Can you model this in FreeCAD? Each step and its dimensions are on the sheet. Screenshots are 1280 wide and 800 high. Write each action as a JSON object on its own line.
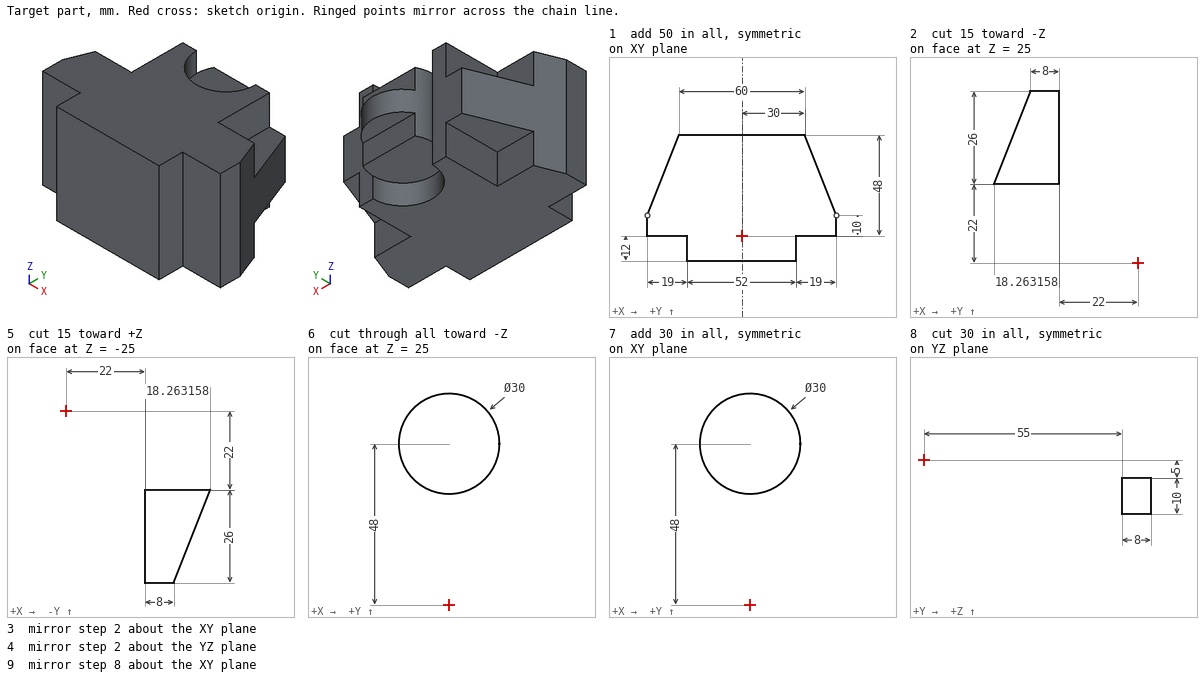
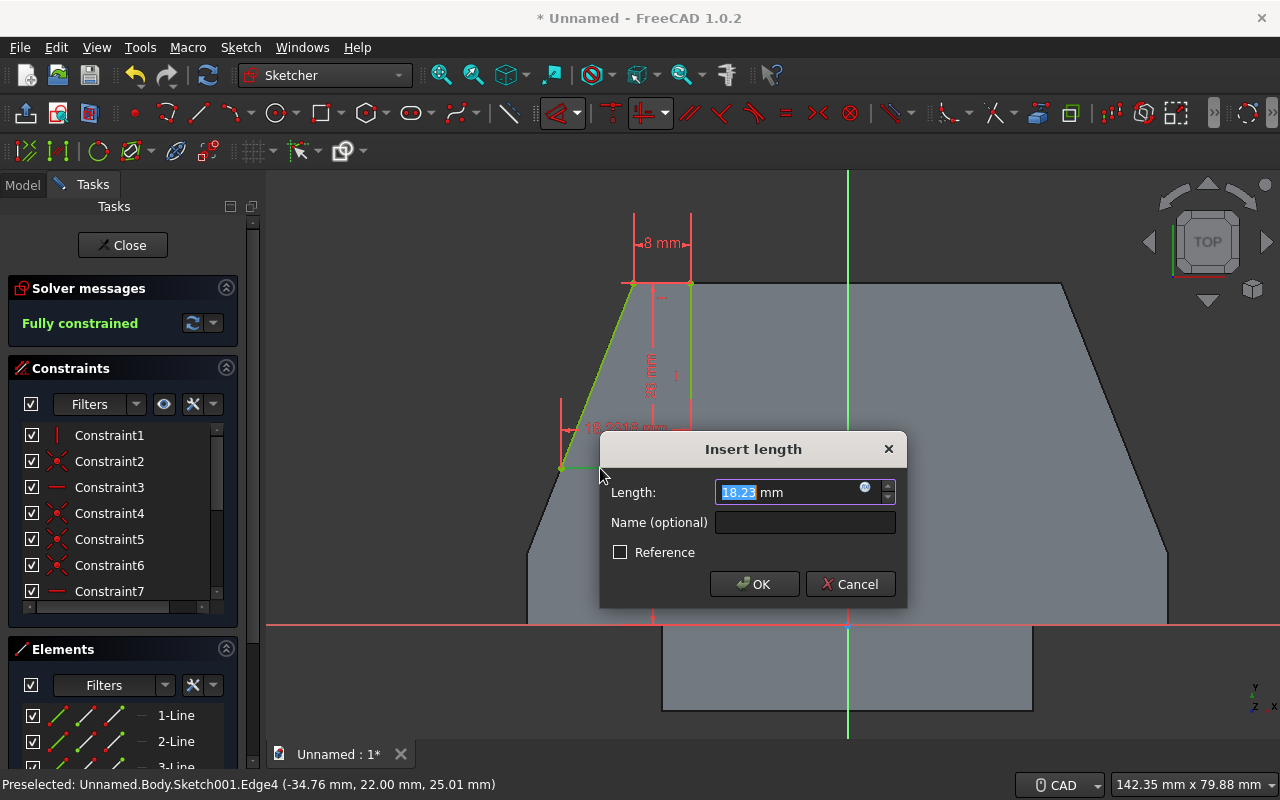
{"action": "type", "text": "18.263158"}
{"action": "key", "text": "Return"}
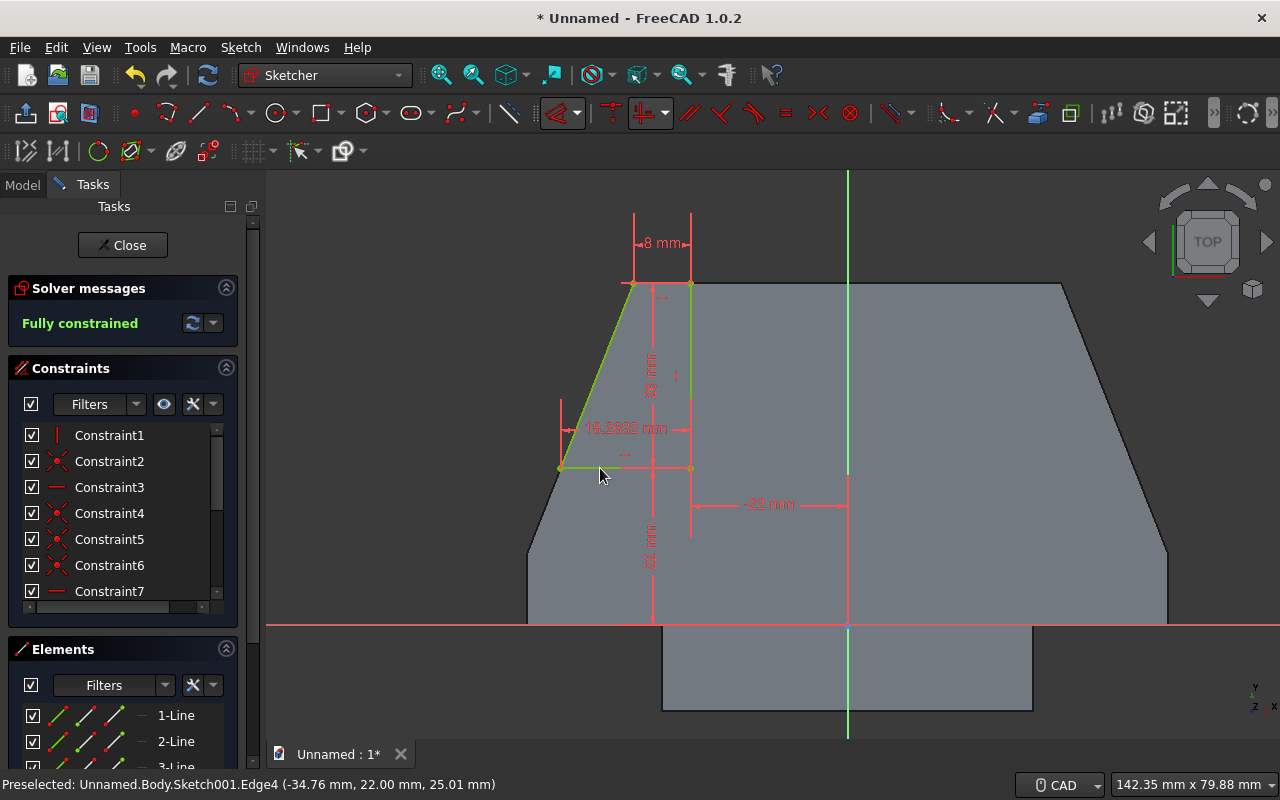
{"action": "left_click", "coordinate": [123, 245]}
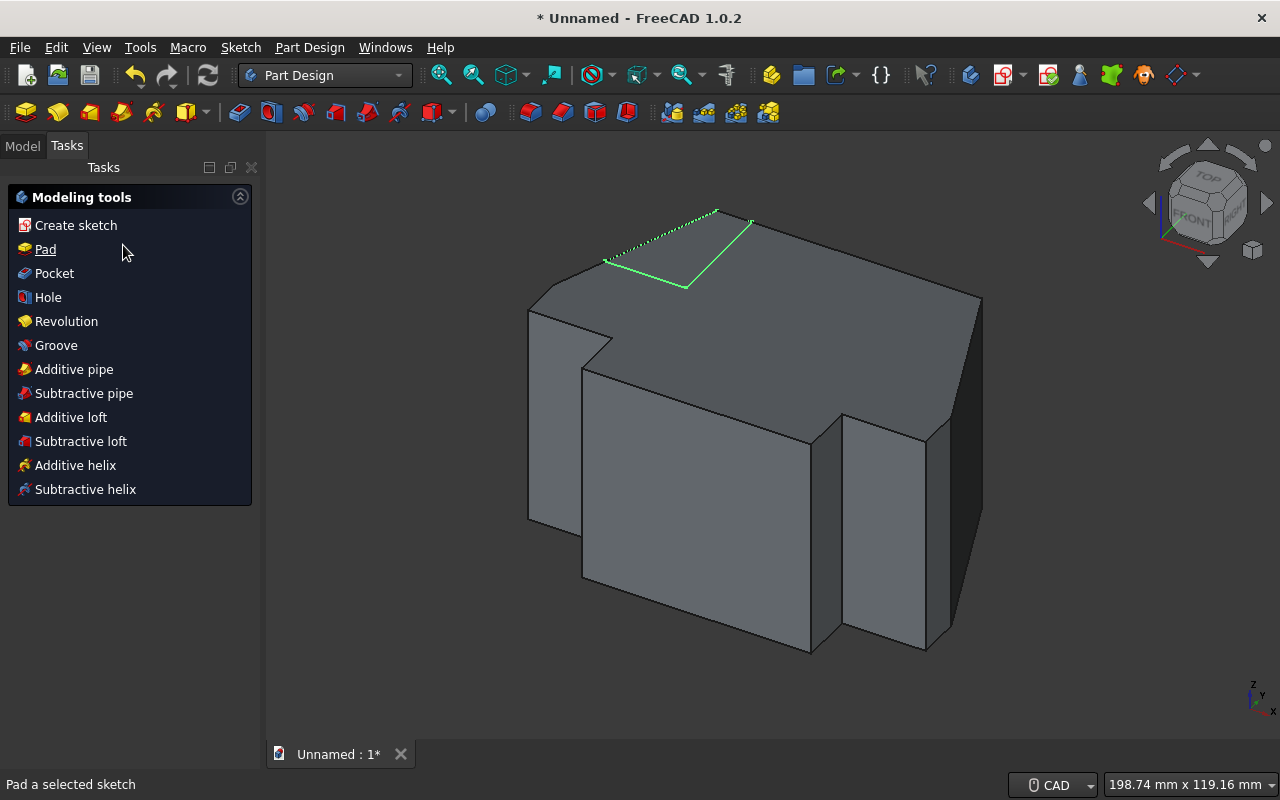
{"action": "left_click", "coordinate": [240, 112]}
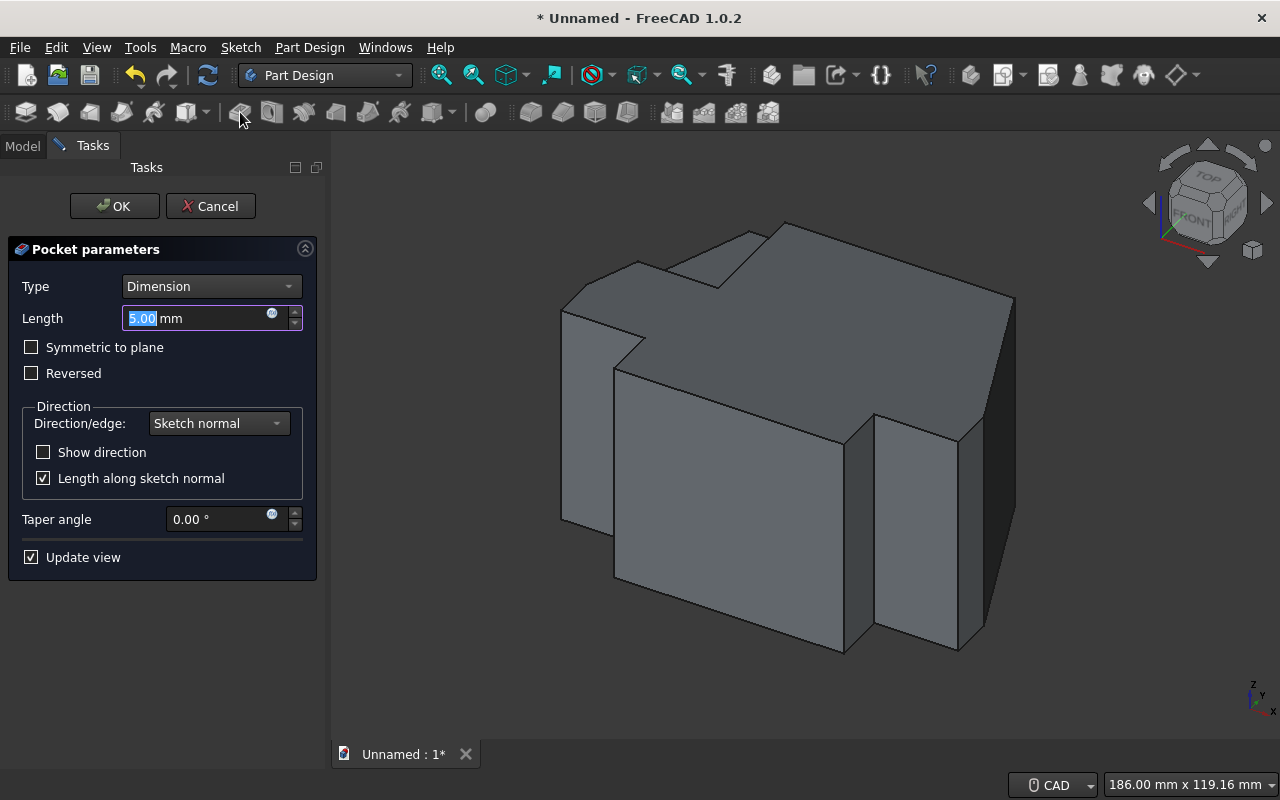
{"action": "type", "text": "15"}
{"action": "key", "text": "Tab"}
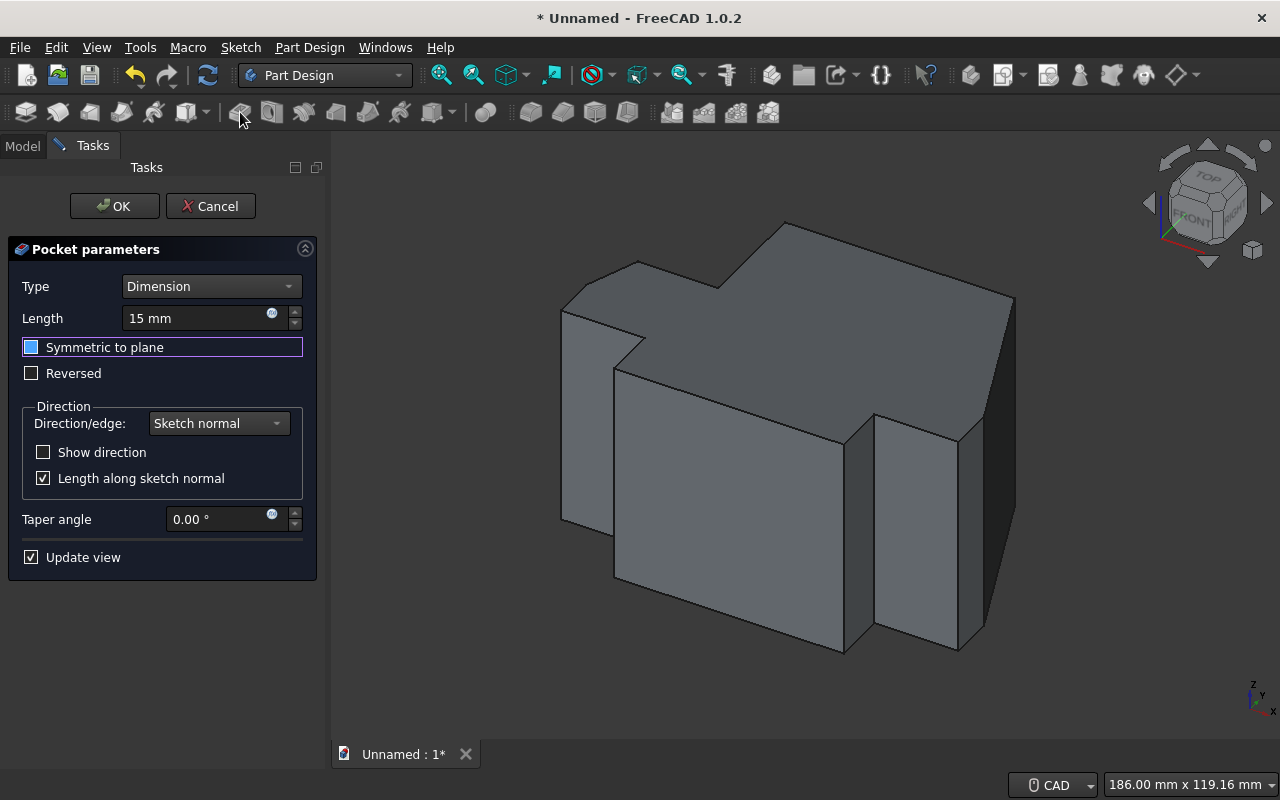
{"action": "left_click", "coordinate": [115, 206]}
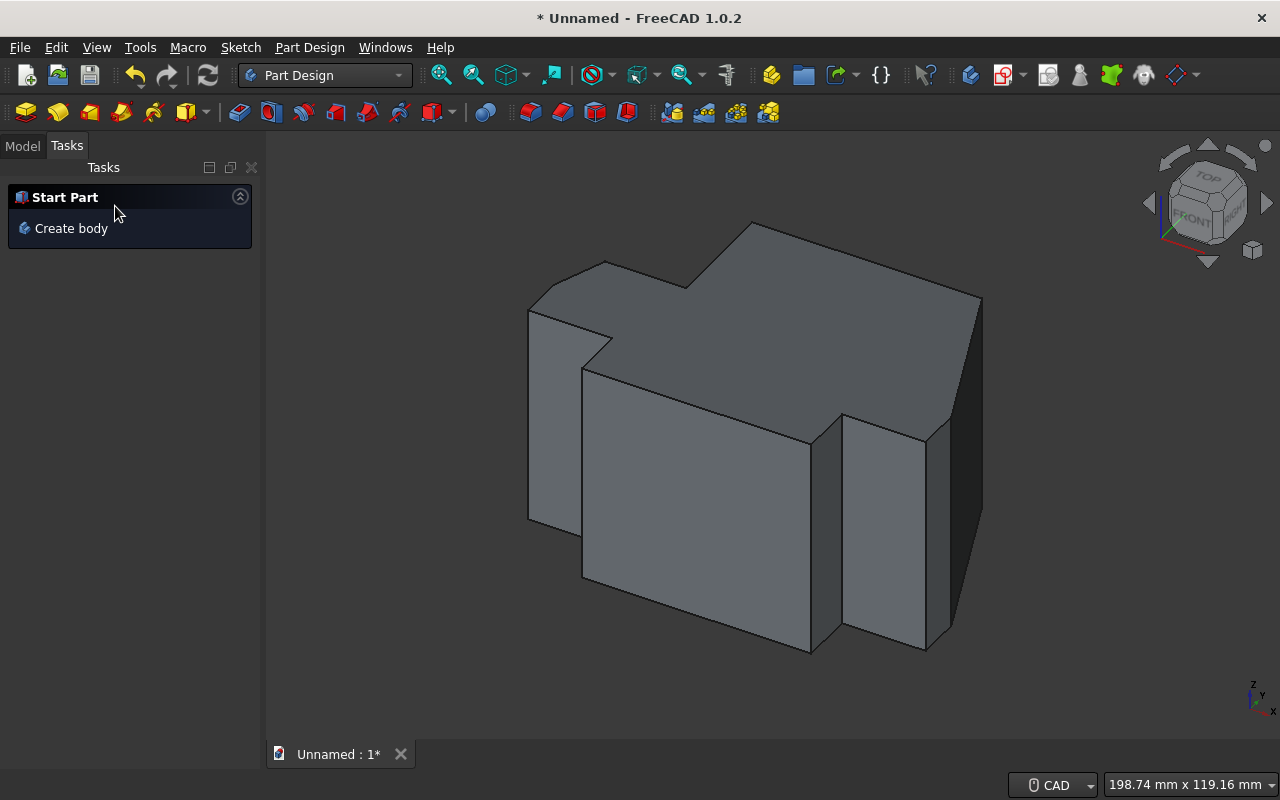
{"action": "left_click", "coordinate": [23, 145]}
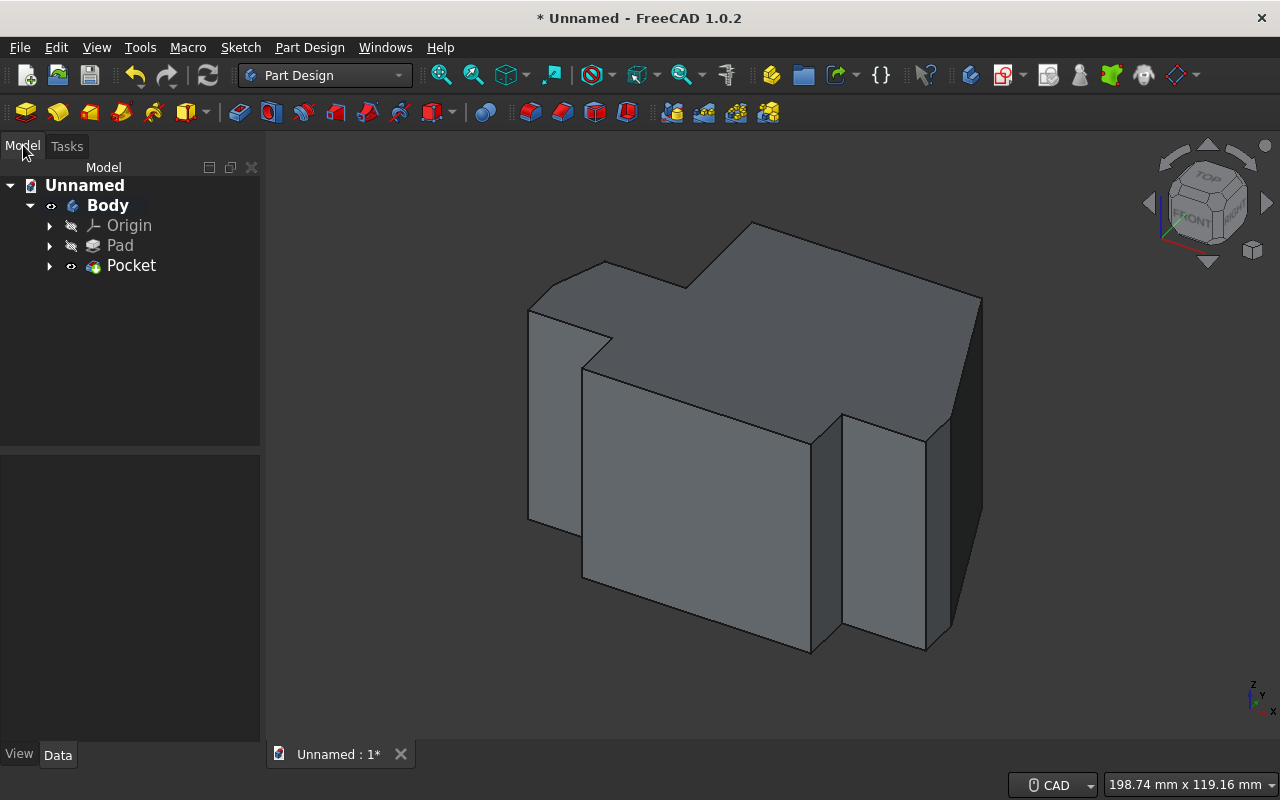
{"action": "left_click", "coordinate": [116, 266]}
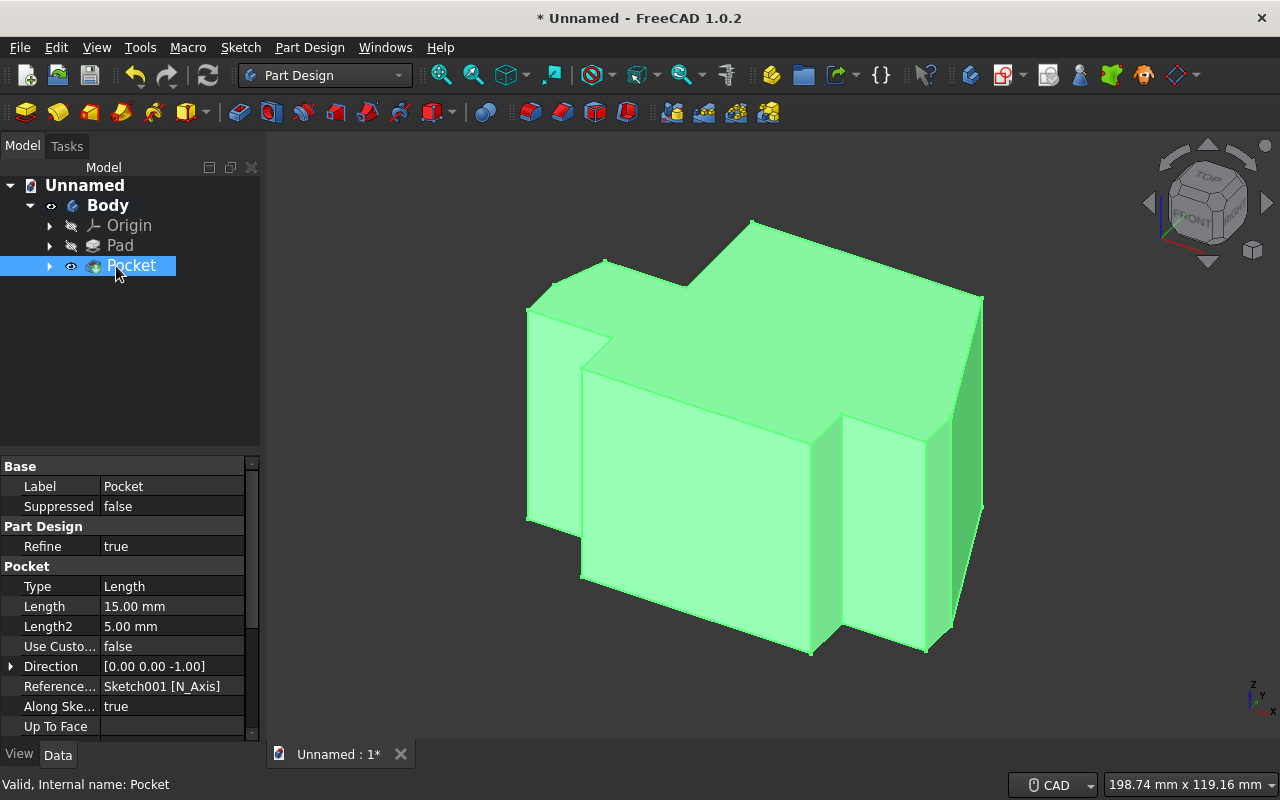
{"action": "left_click", "coordinate": [672, 112]}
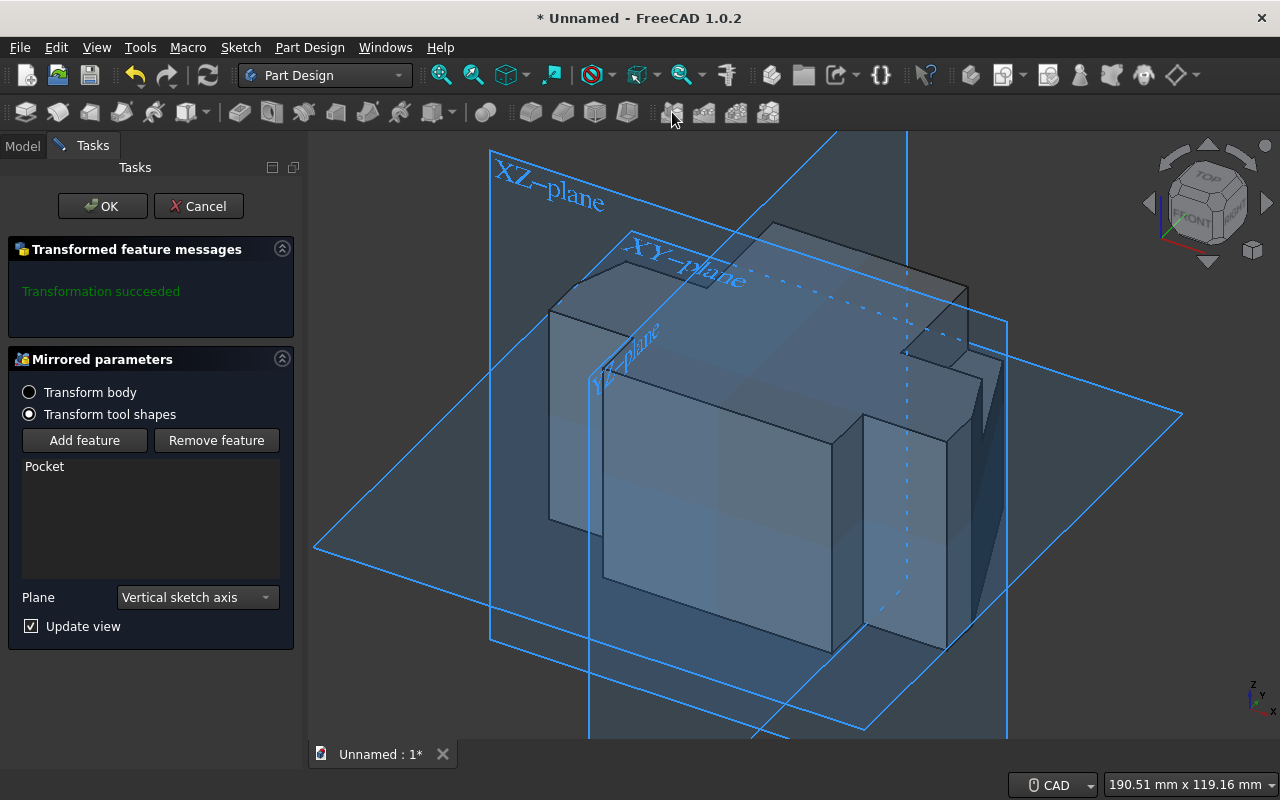
{"action": "left_click", "coordinate": [198, 598]}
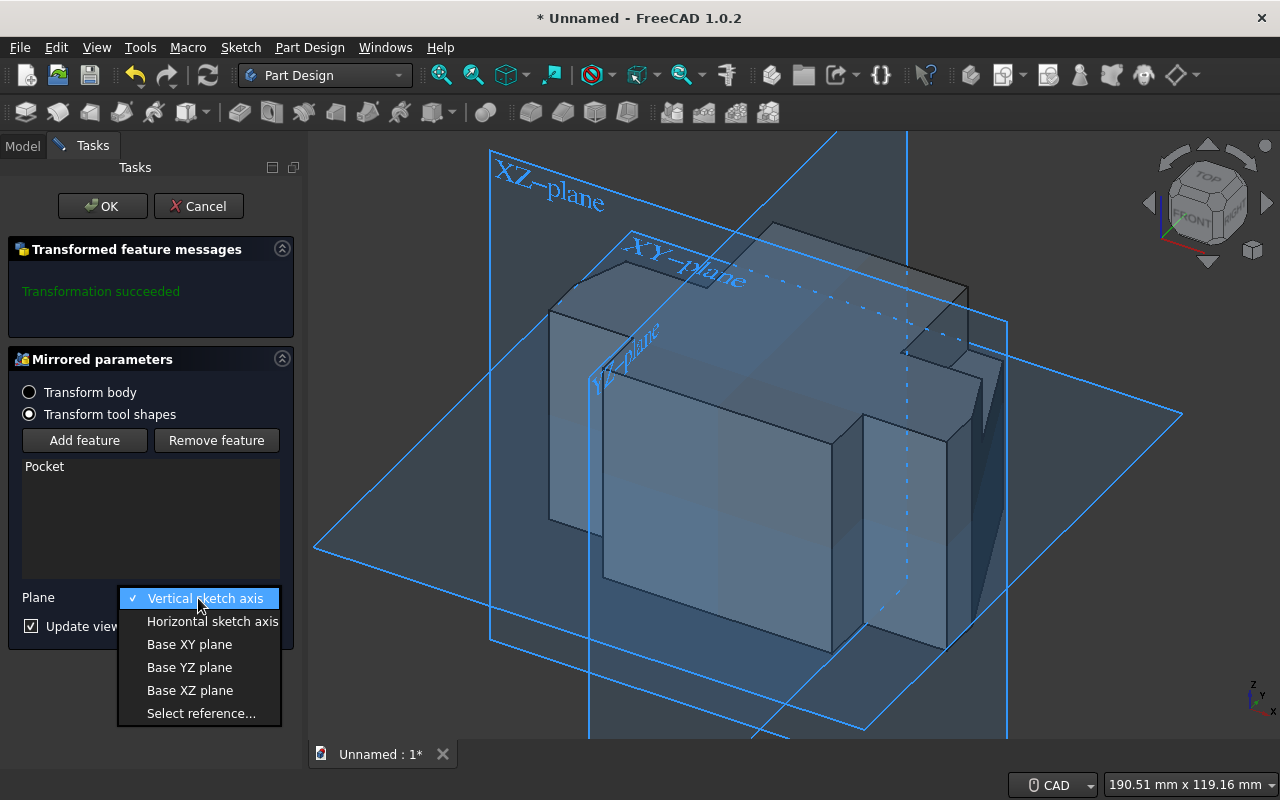
{"action": "left_click", "coordinate": [198, 644]}